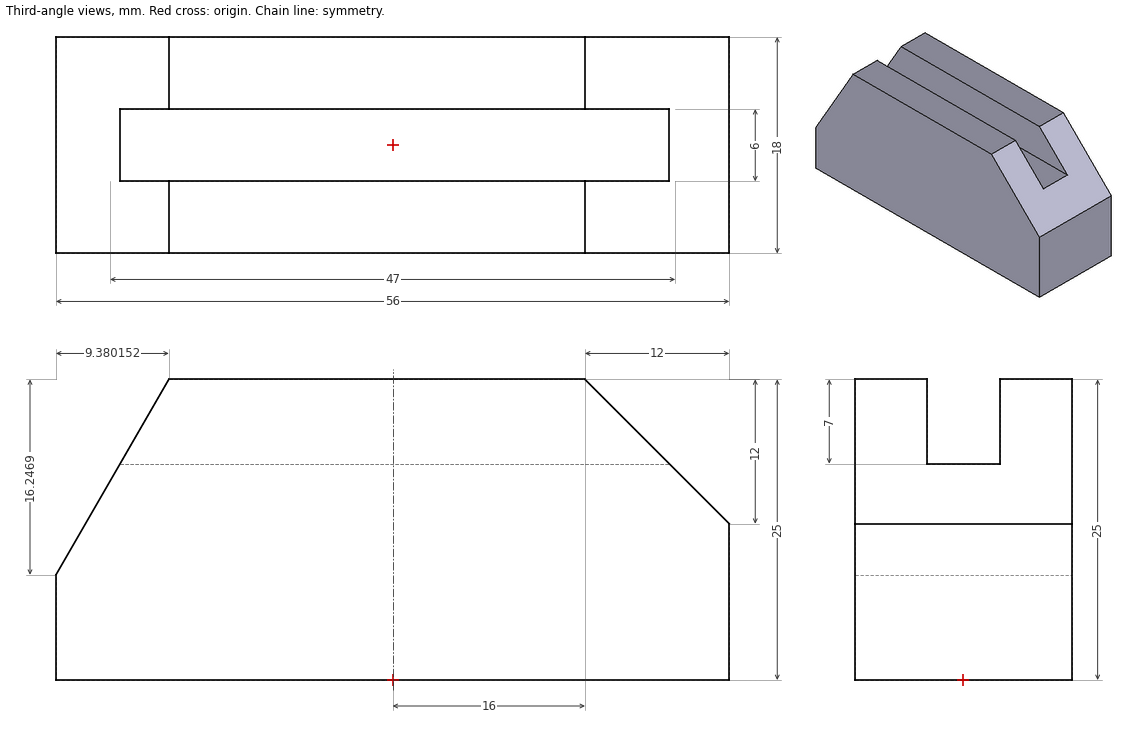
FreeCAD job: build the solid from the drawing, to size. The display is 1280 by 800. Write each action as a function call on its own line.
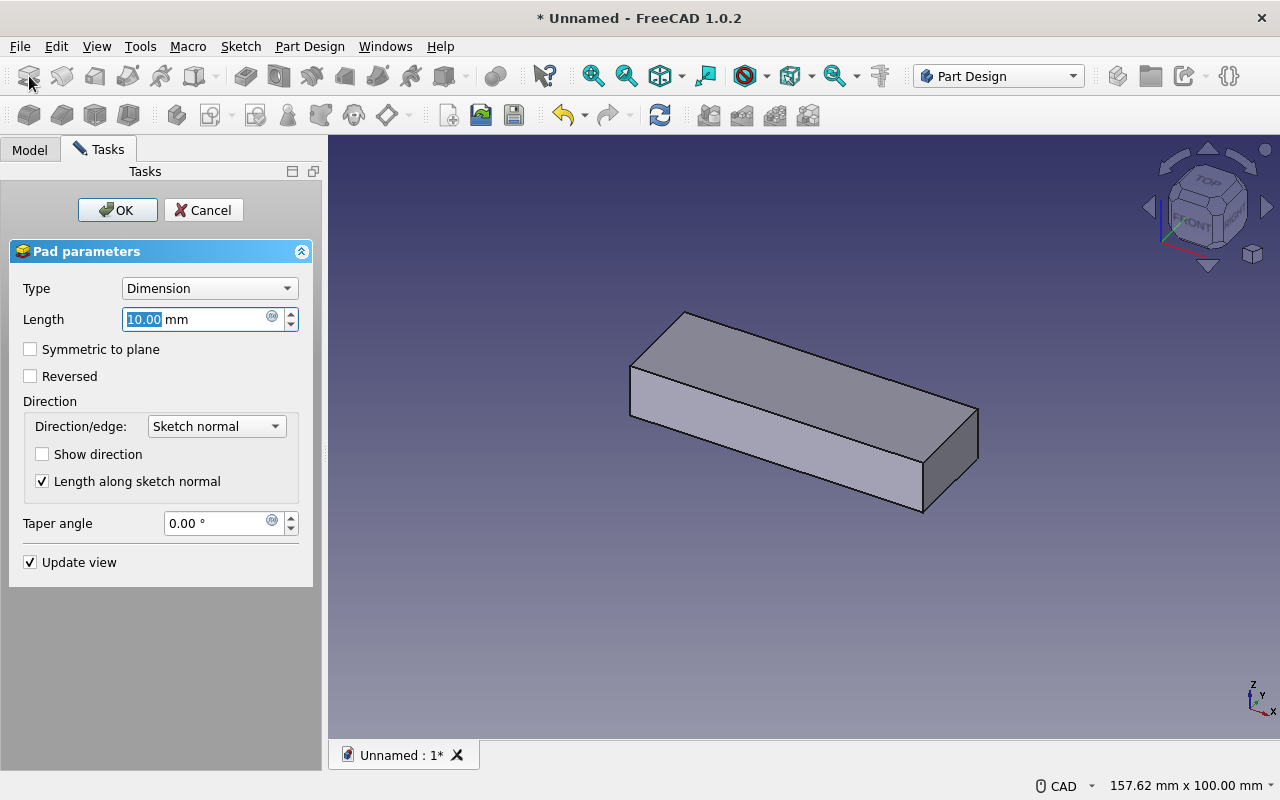
text(25)
key(Tab)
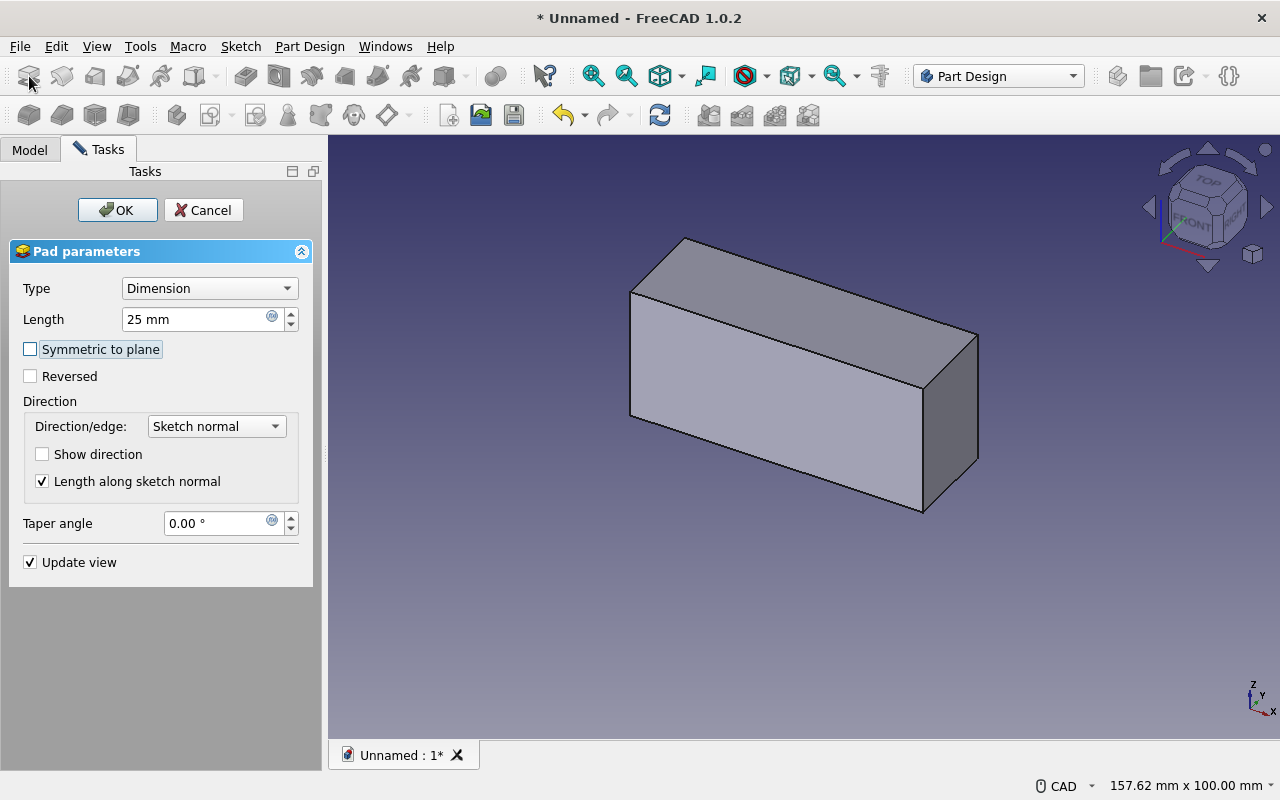
click(118, 210)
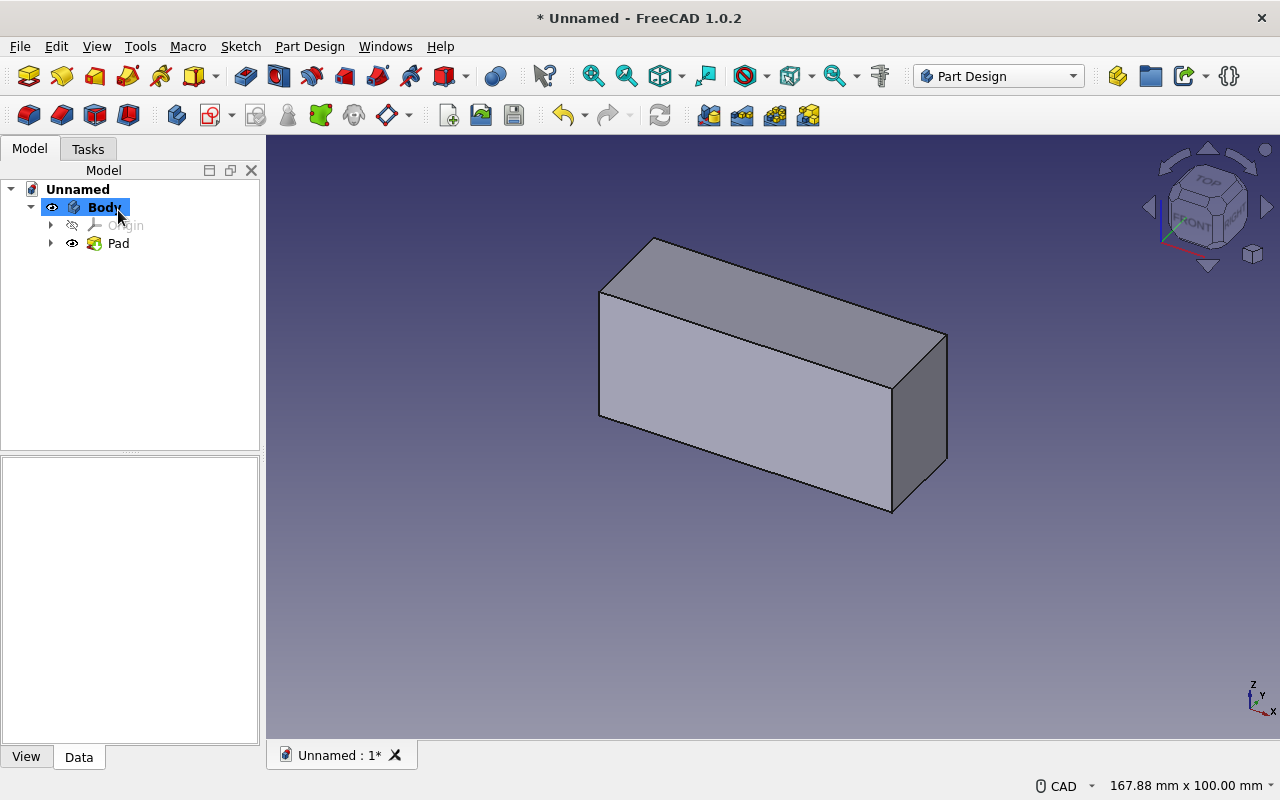
click(788, 415)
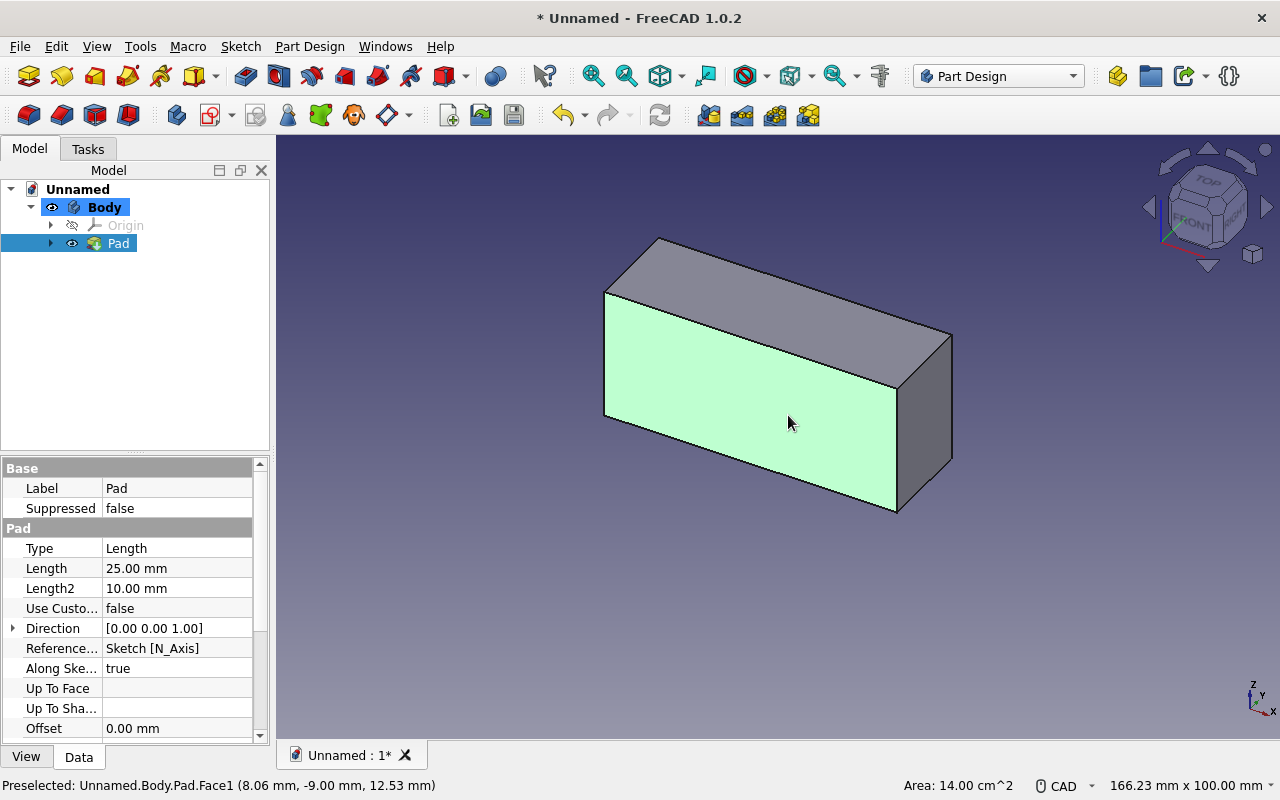
click(210, 116)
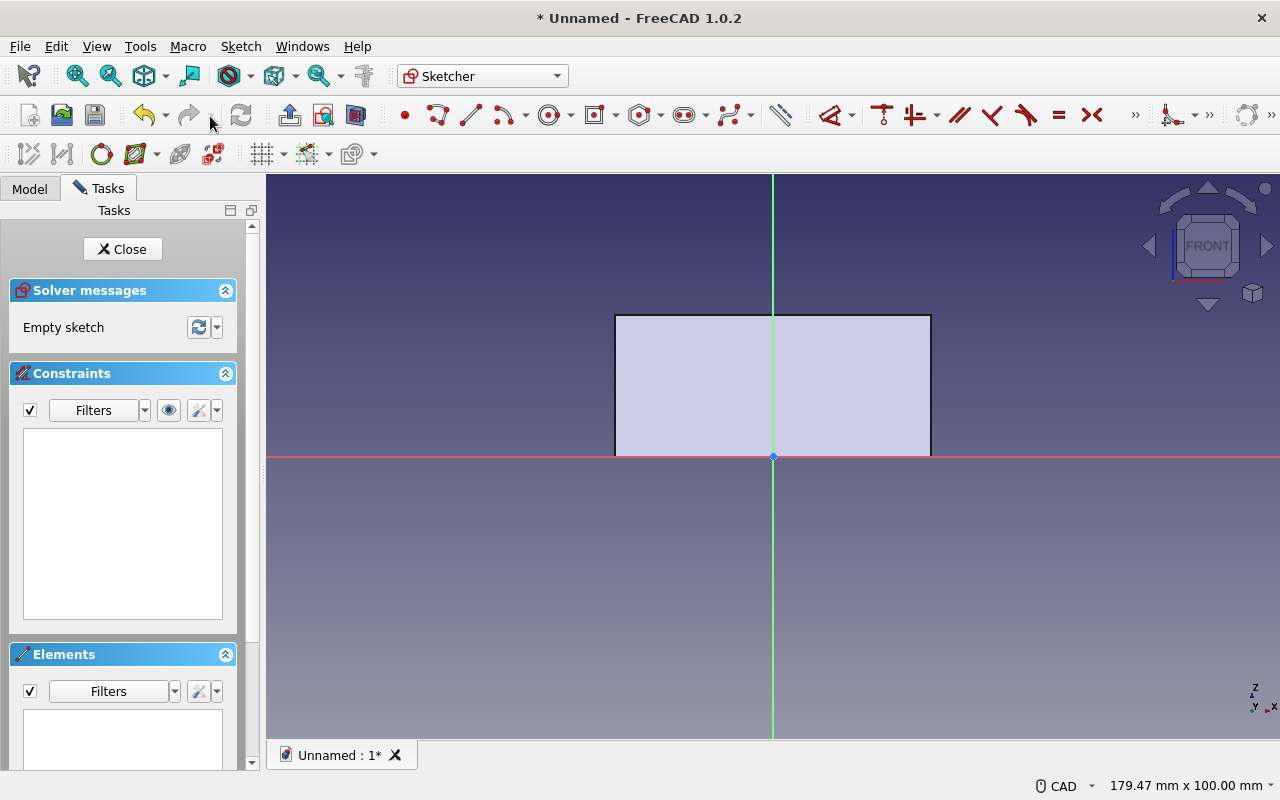
scroll(856, 300, up, 3)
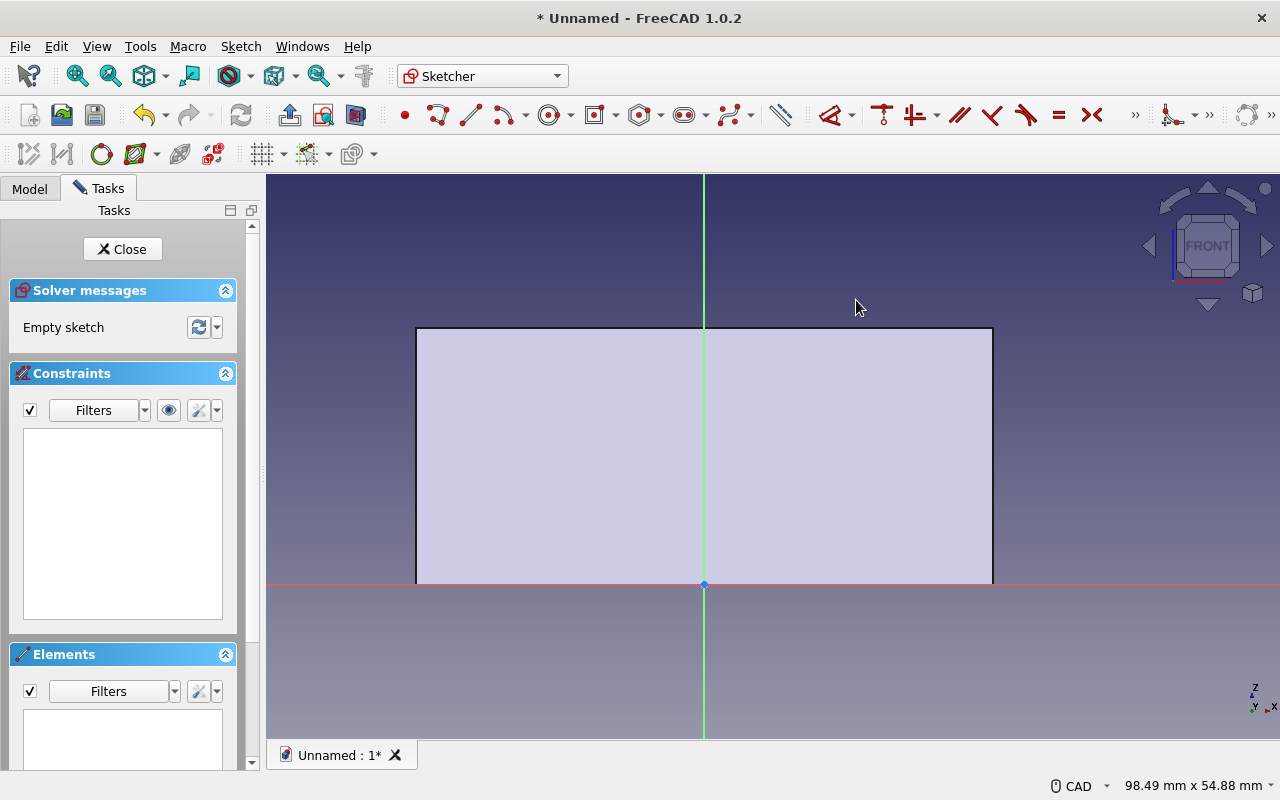
click(438, 116)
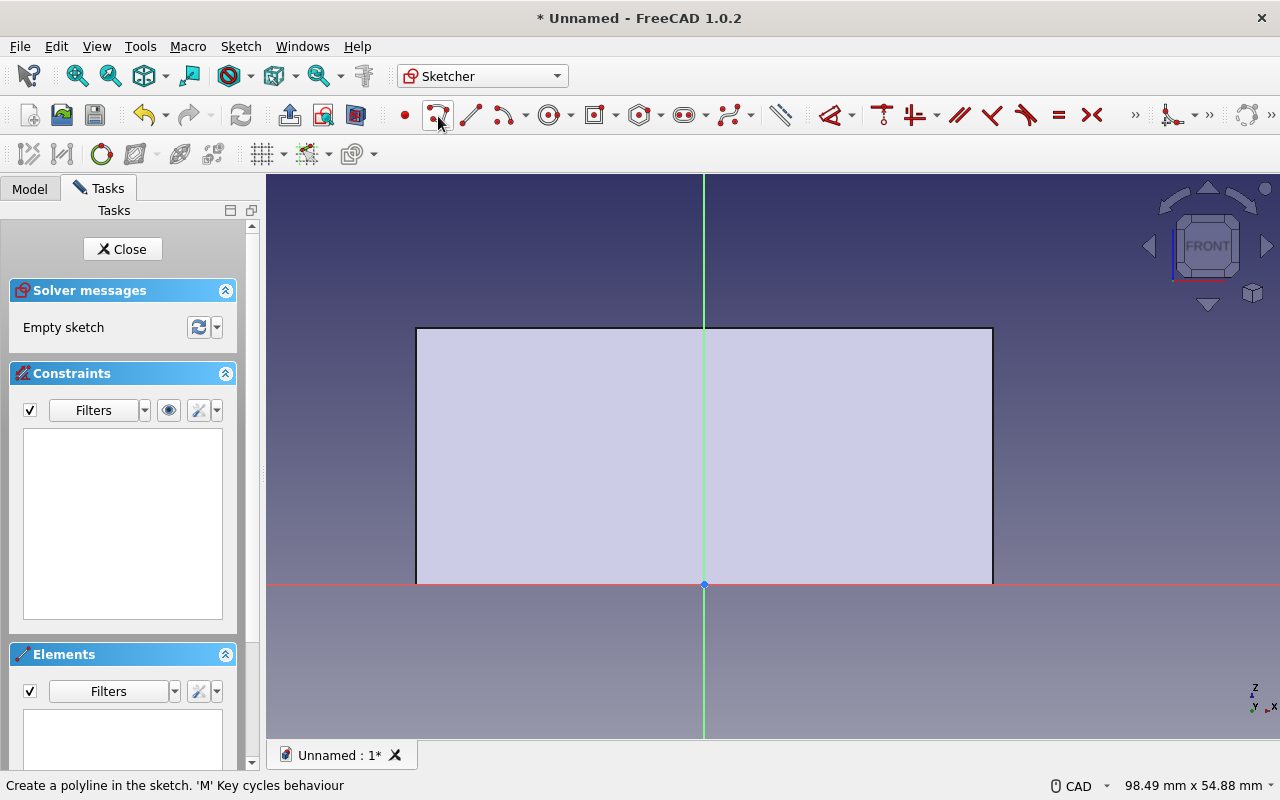
click(869, 328)
click(993, 451)
click(993, 328)
click(869, 329)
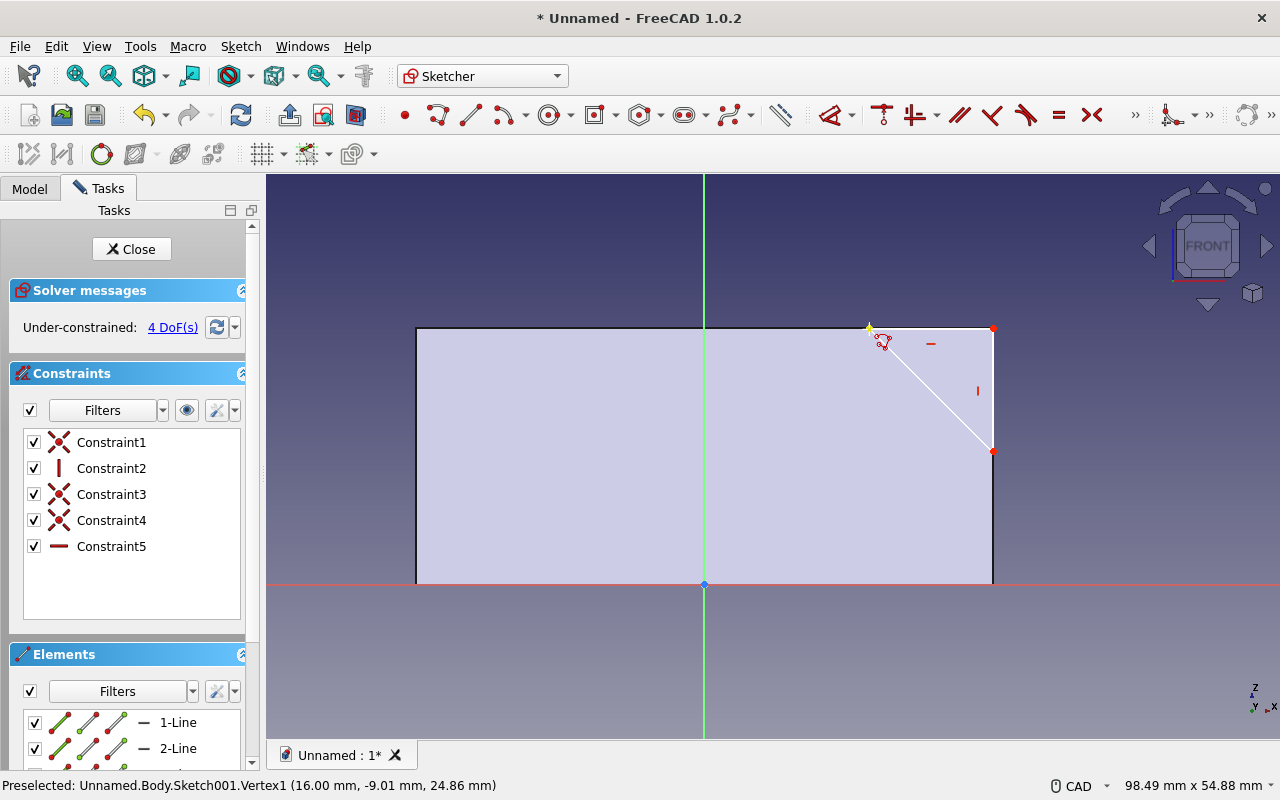
click(416, 495)
click(513, 328)
click(416, 328)
click(416, 496)
key(Escape)
key(Escape)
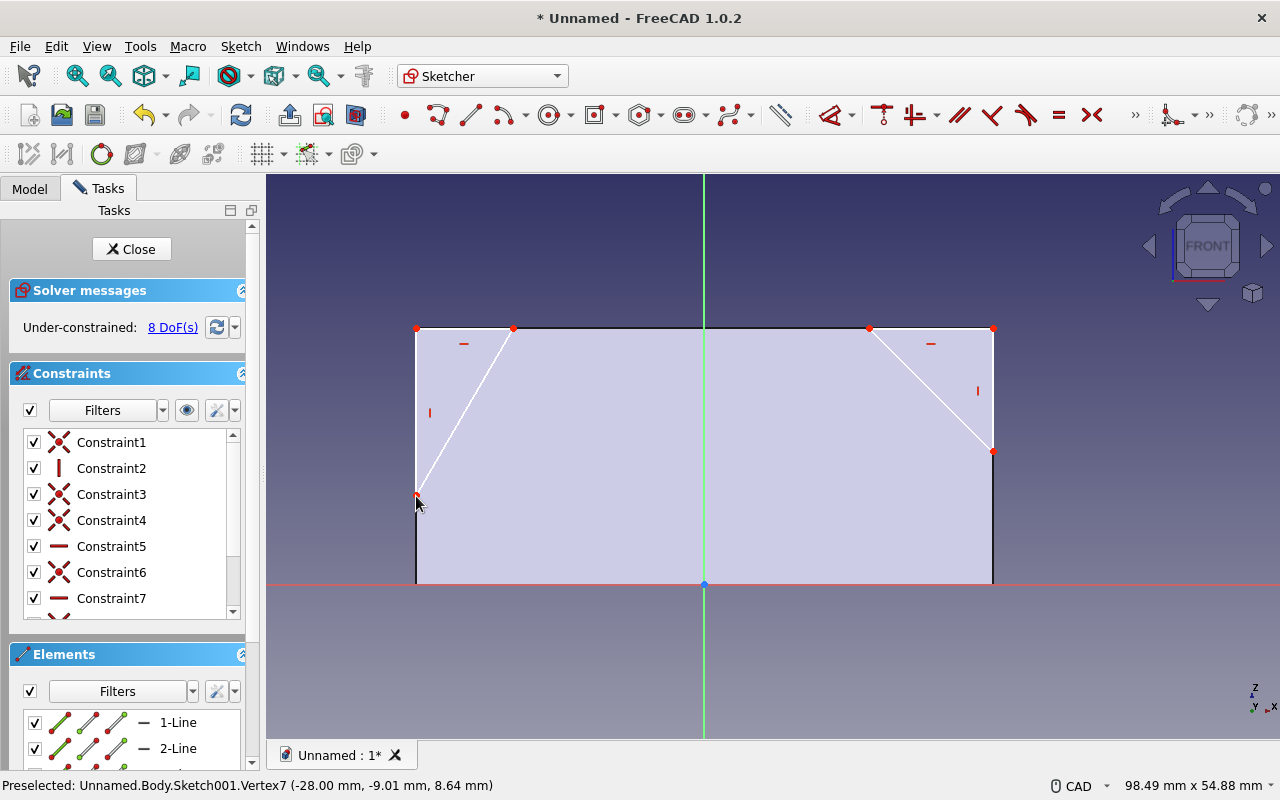
click(993, 329)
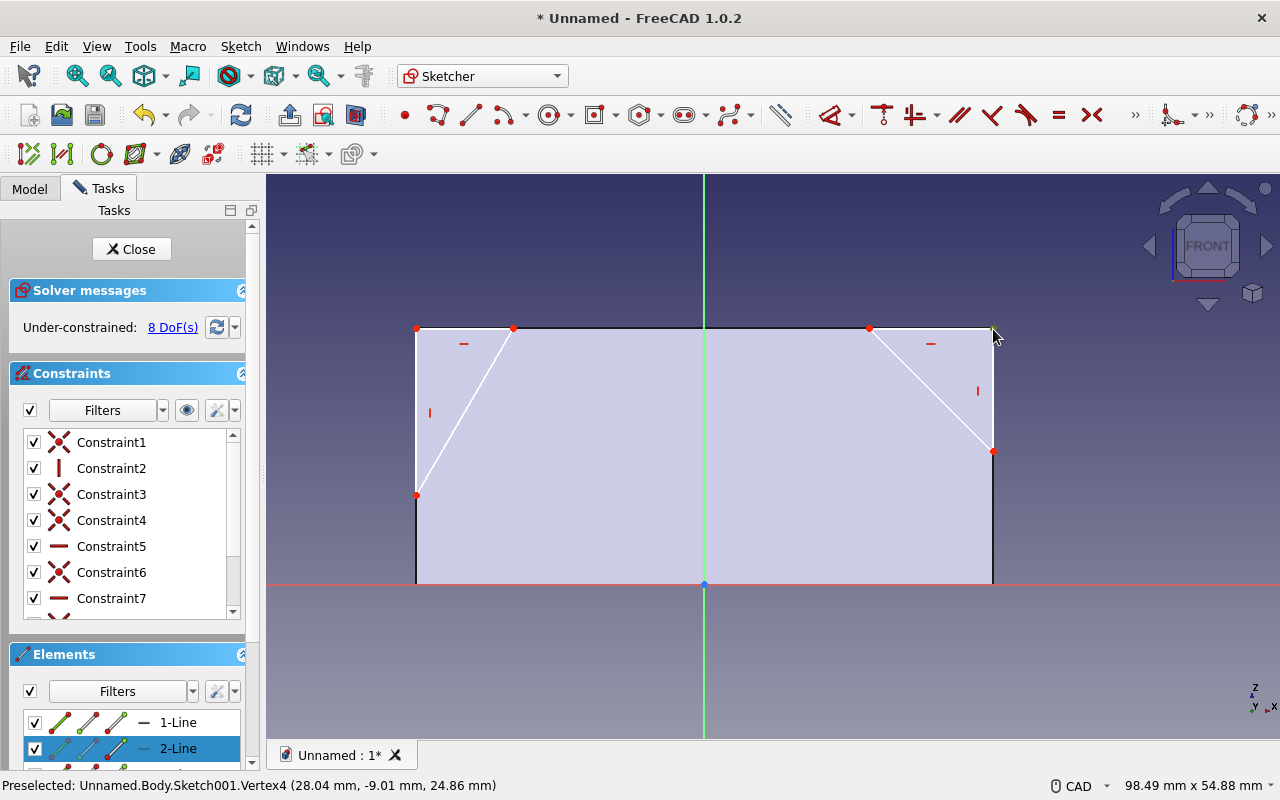
click(416, 329)